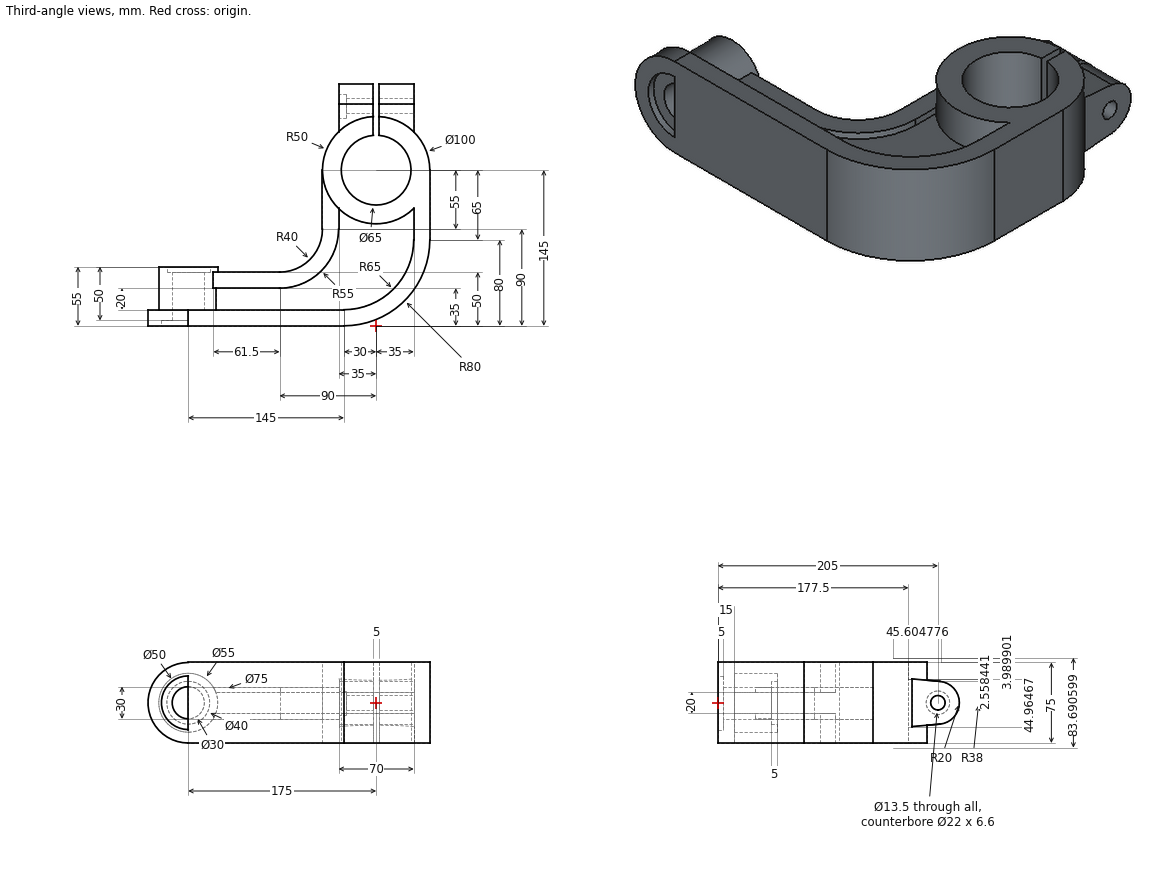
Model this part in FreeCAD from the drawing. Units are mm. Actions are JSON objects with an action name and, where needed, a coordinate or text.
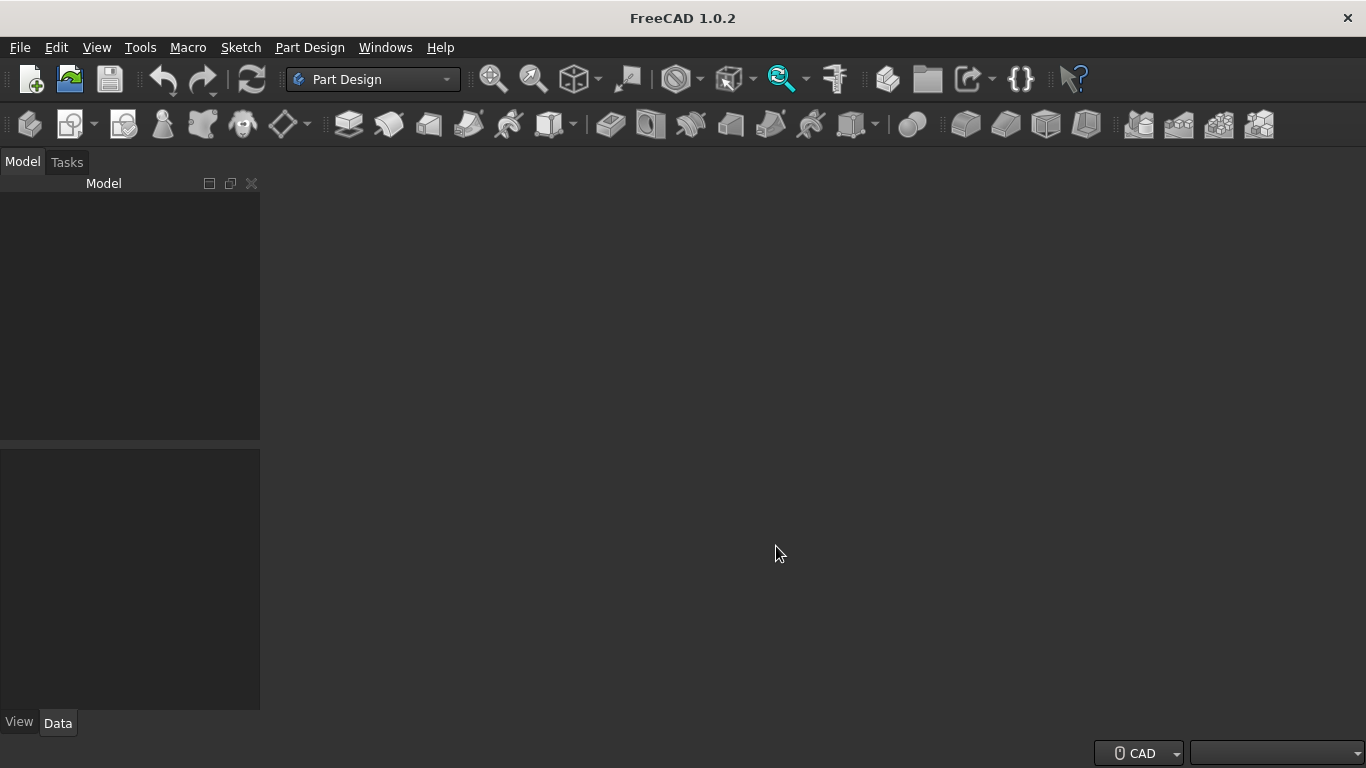
{"action": "key", "text": "ctrl+n"}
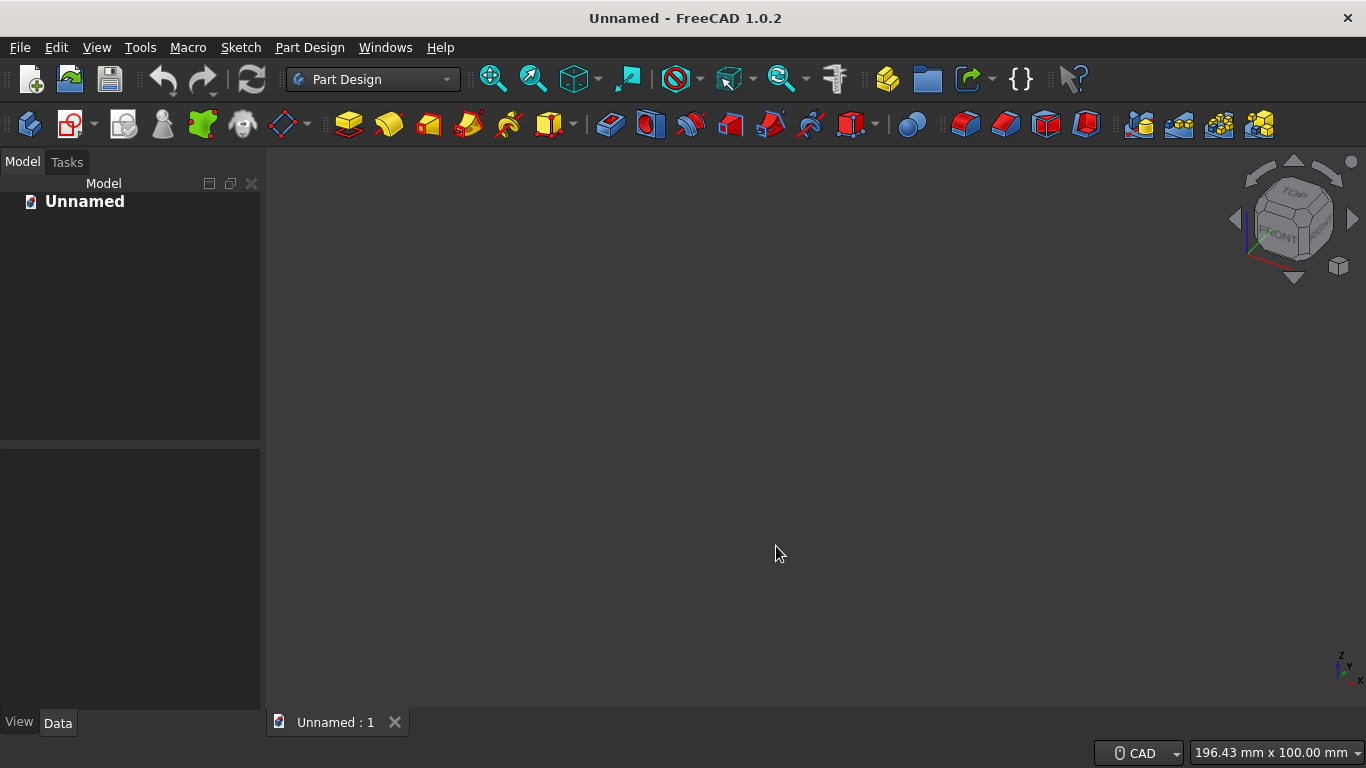
{"action": "left_click", "coordinate": [70, 124]}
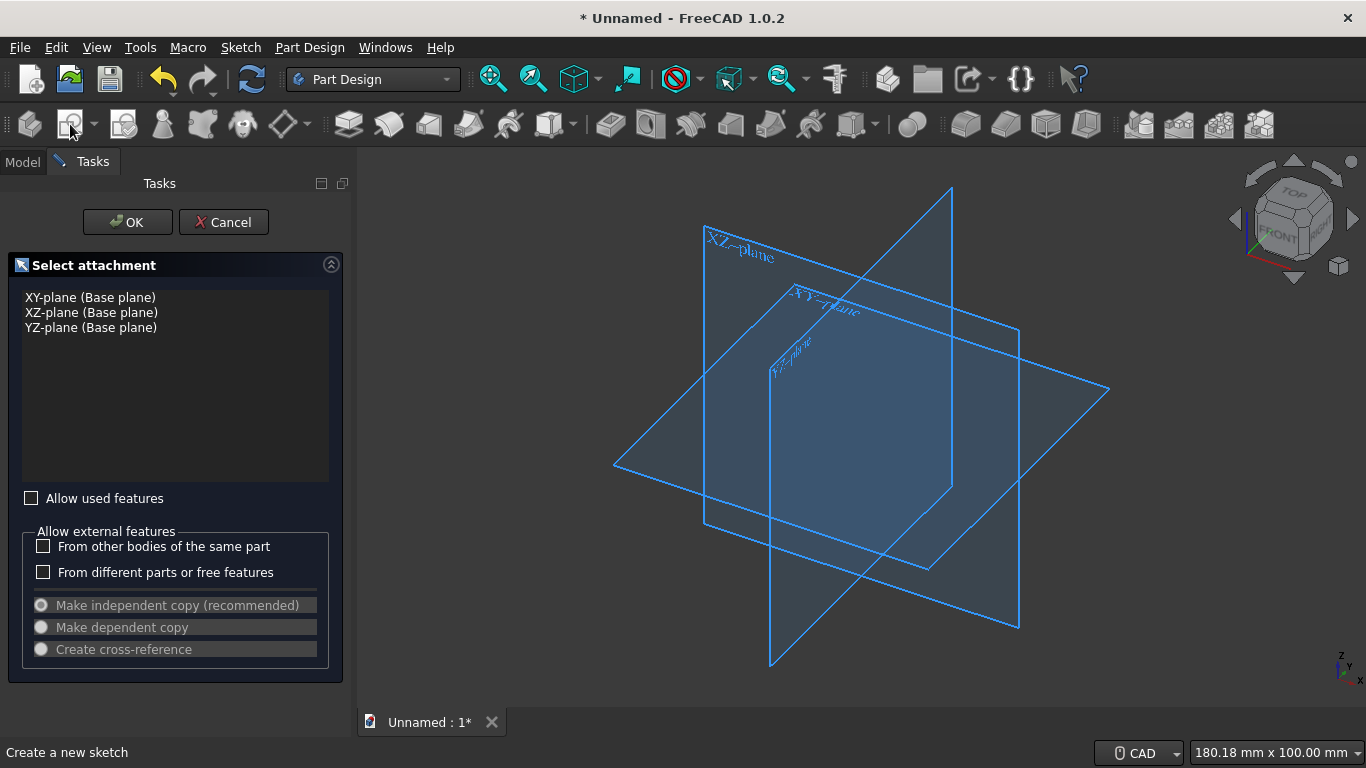
{"action": "left_click", "coordinate": [82, 298]}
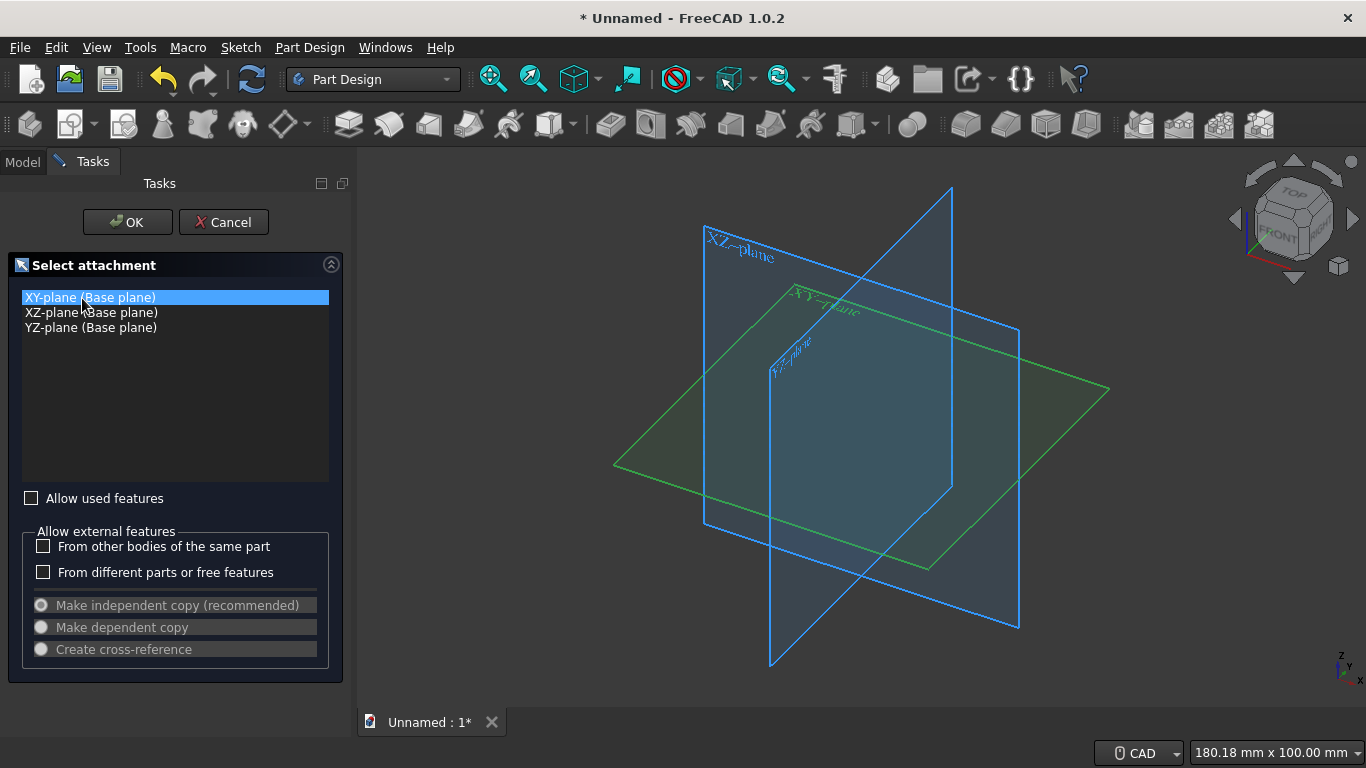
{"action": "left_click", "coordinate": [128, 222]}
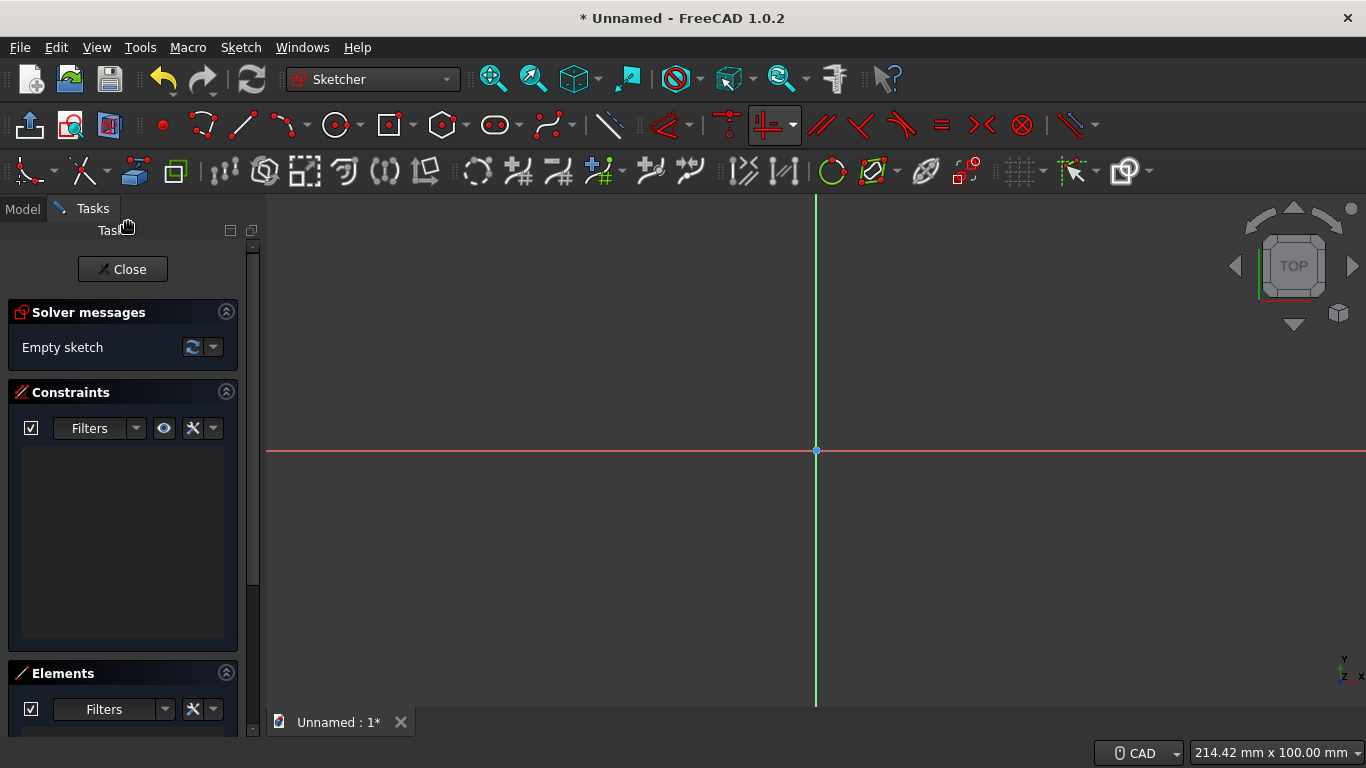
{"action": "scroll", "coordinate": [718, 666], "scroll_direction": "down", "scroll_amount": 6}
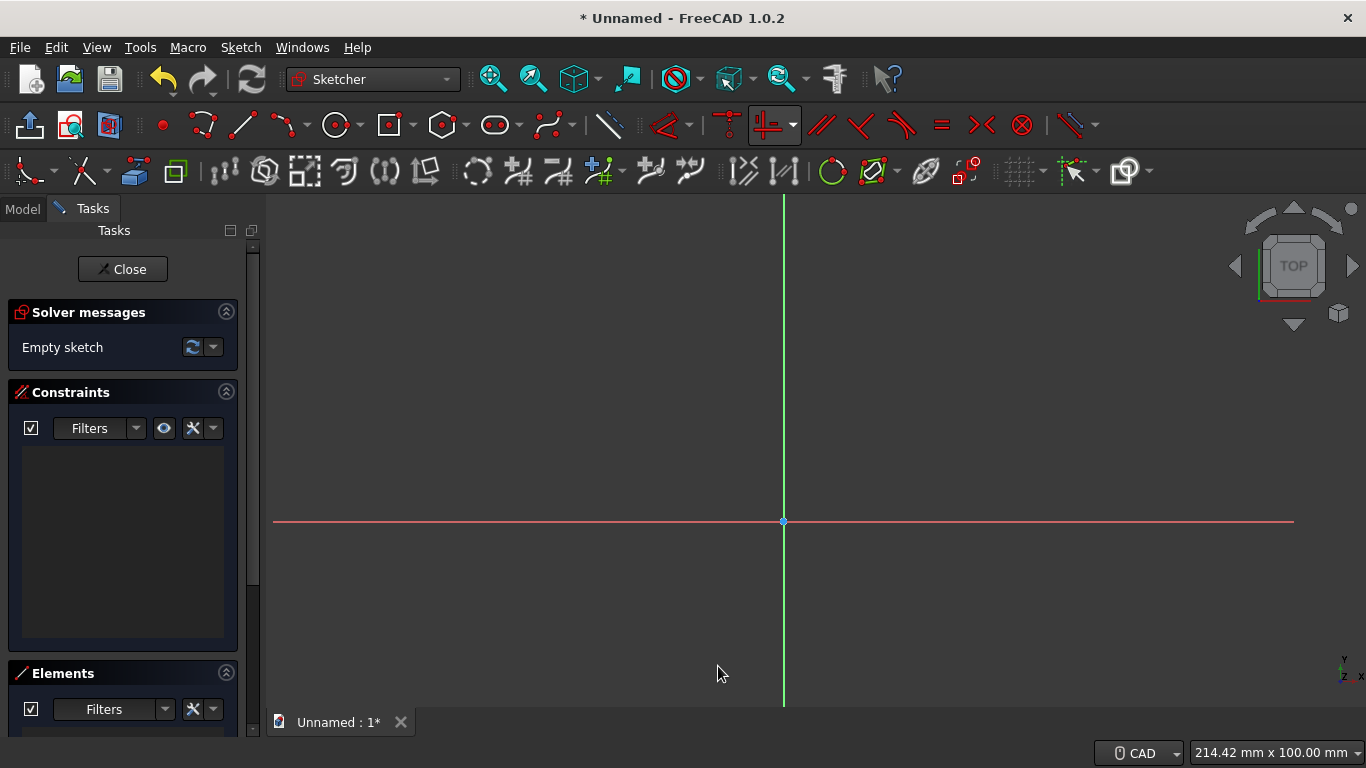
{"action": "left_click", "coordinate": [336, 126]}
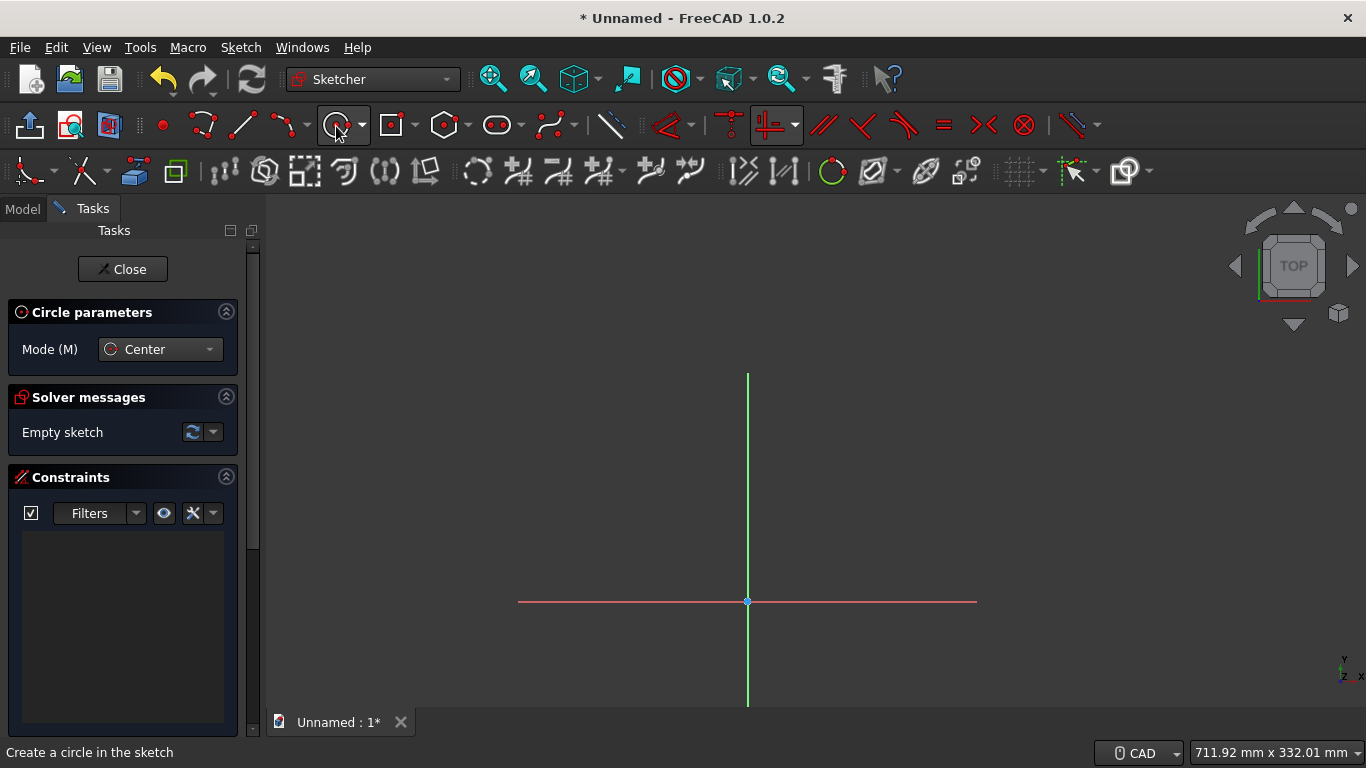
{"action": "left_click", "coordinate": [748, 378]}
{"action": "left_click", "coordinate": [802, 323]}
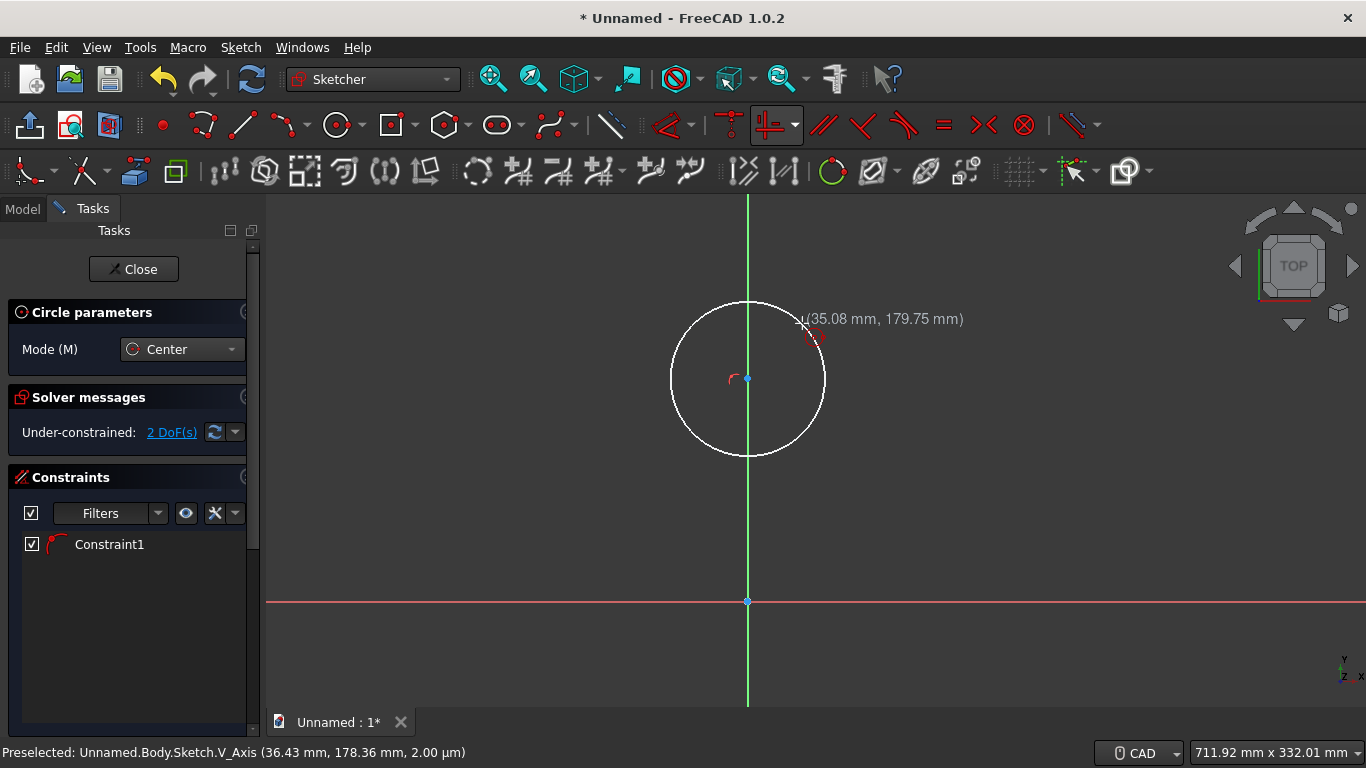
{"action": "left_click", "coordinate": [748, 379]}
{"action": "left_click", "coordinate": [783, 342]}
{"action": "key", "text": "Escape"}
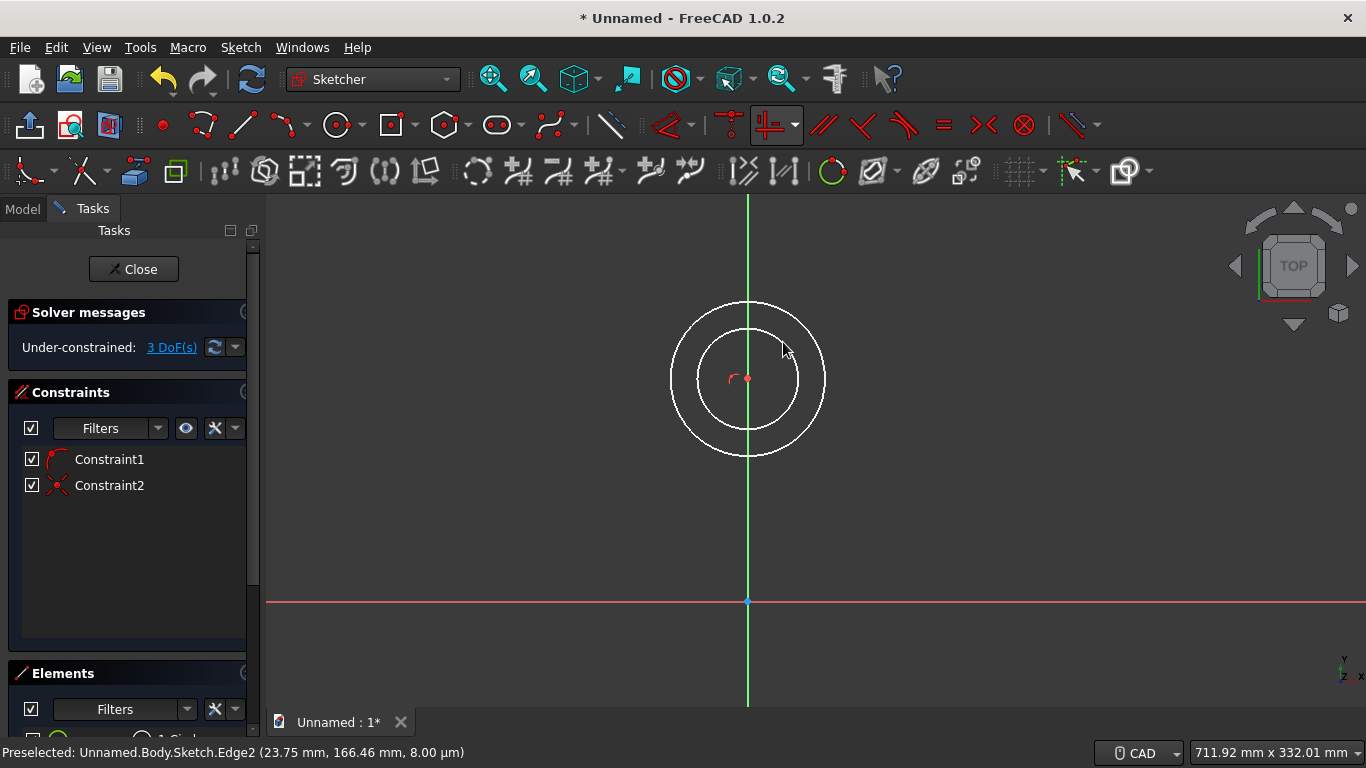
{"action": "left_click", "coordinate": [666, 126]}